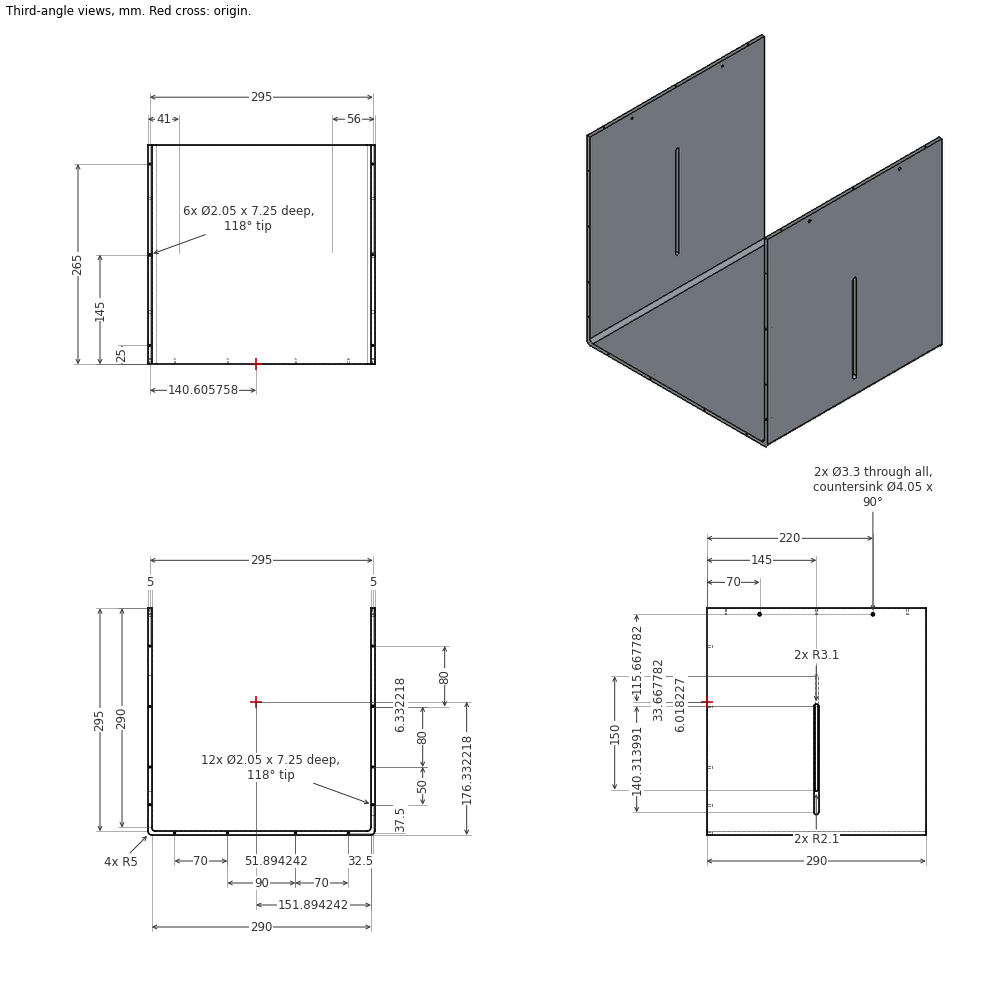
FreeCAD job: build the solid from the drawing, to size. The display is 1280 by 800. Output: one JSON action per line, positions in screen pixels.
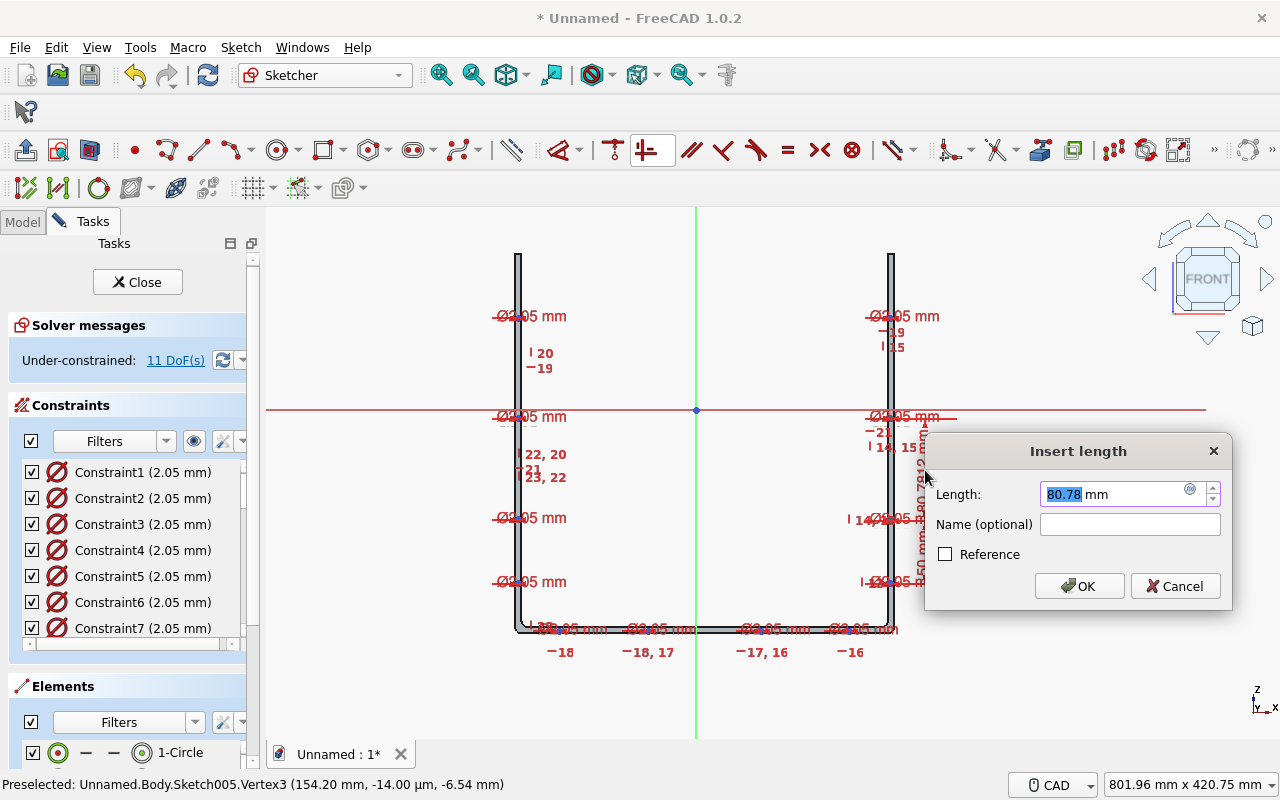
{"action": "type", "text": "80"}
{"action": "key", "text": "Return"}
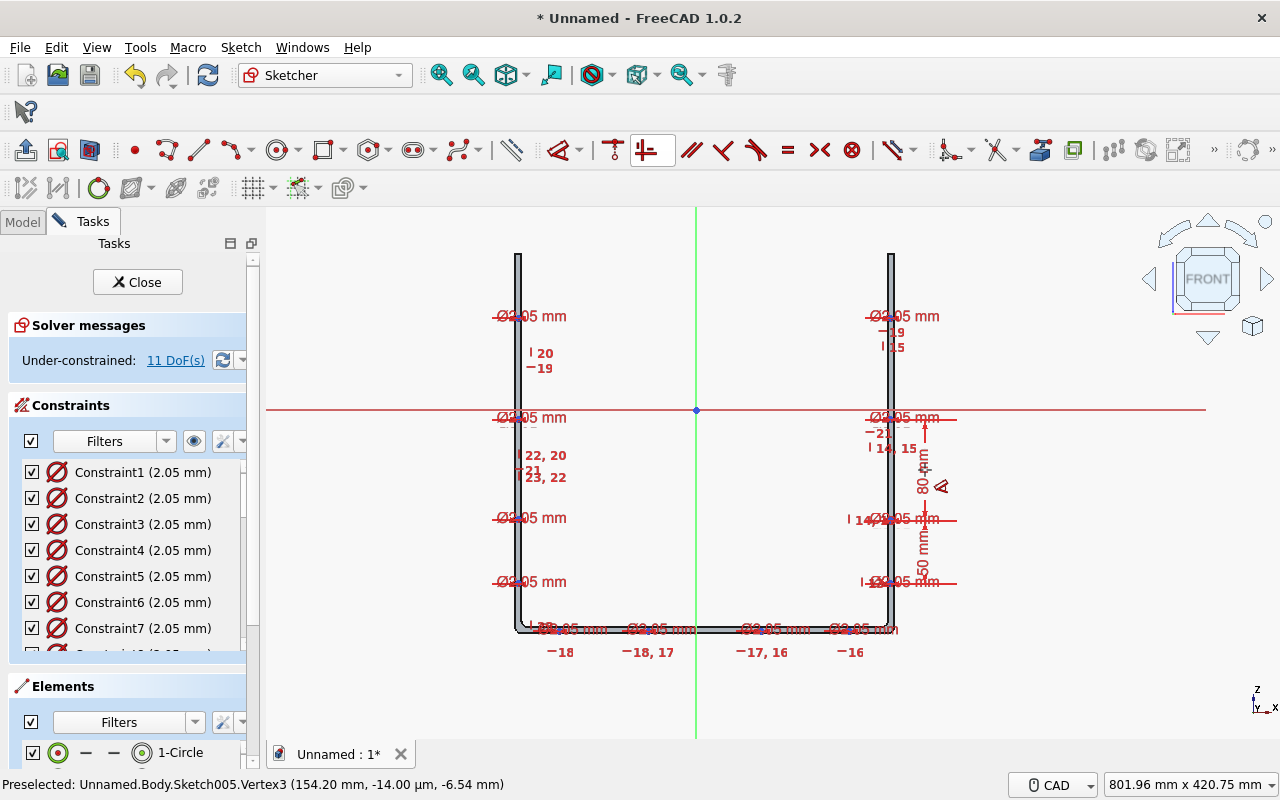
{"action": "left_click", "coordinate": [891, 420]}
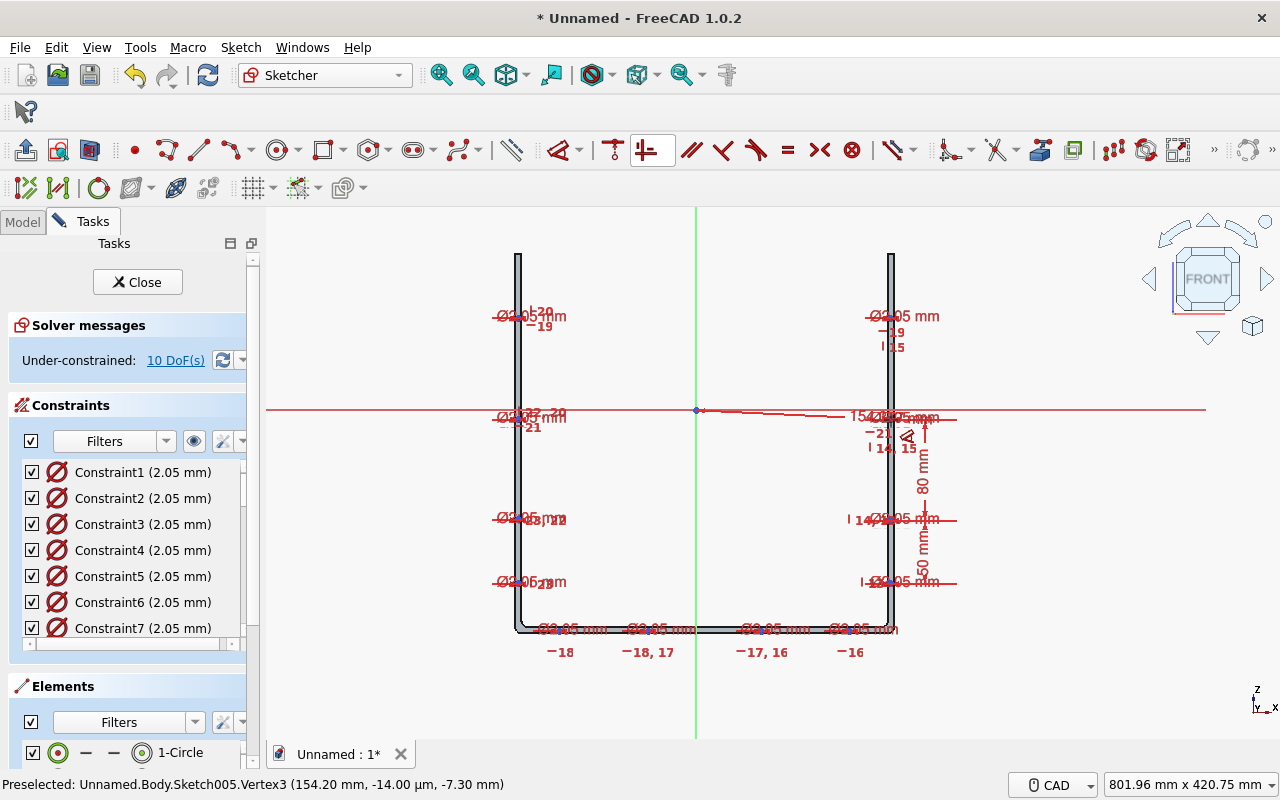
{"action": "left_click", "coordinate": [891, 318]}
{"action": "left_click", "coordinate": [925, 369]}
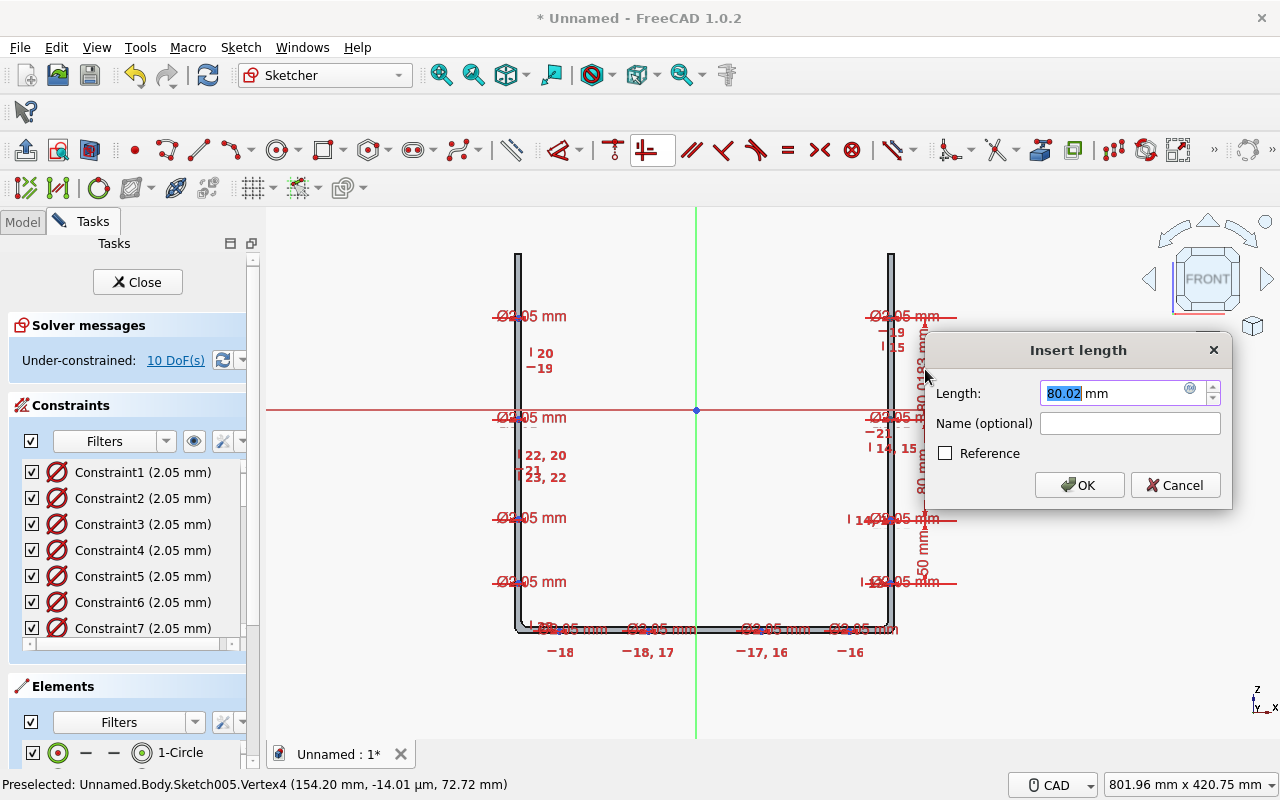
{"action": "type", "text": "80"}
{"action": "key", "text": "Return"}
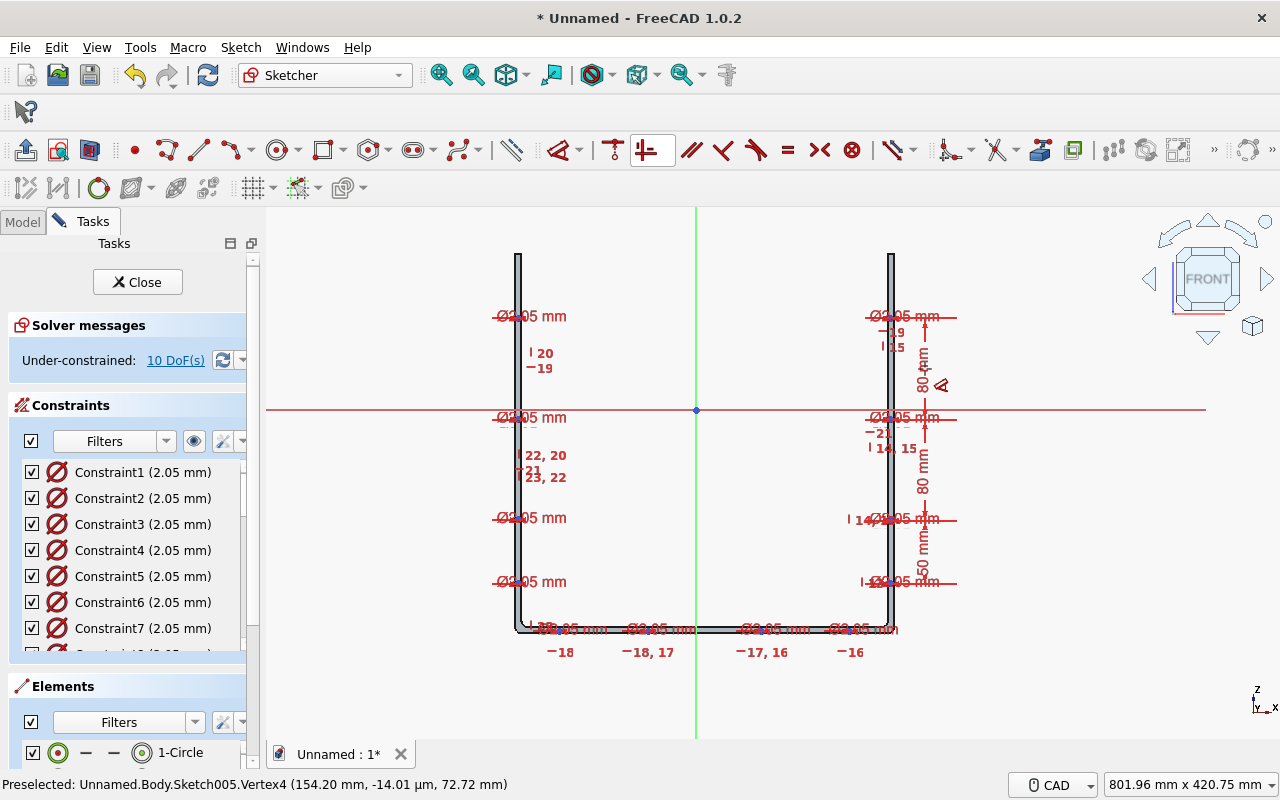
{"action": "left_click", "coordinate": [850, 631]}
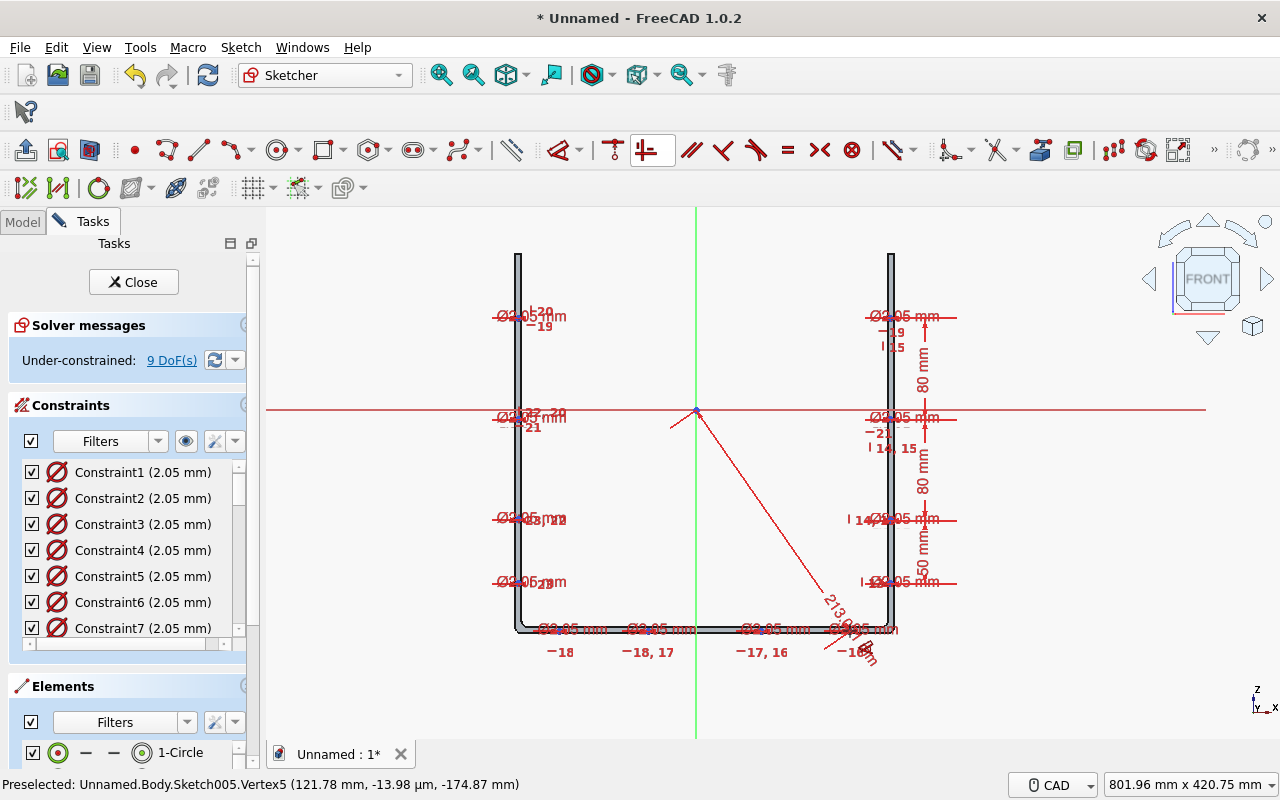
{"action": "left_click", "coordinate": [762, 631]}
{"action": "left_click", "coordinate": [806, 665]}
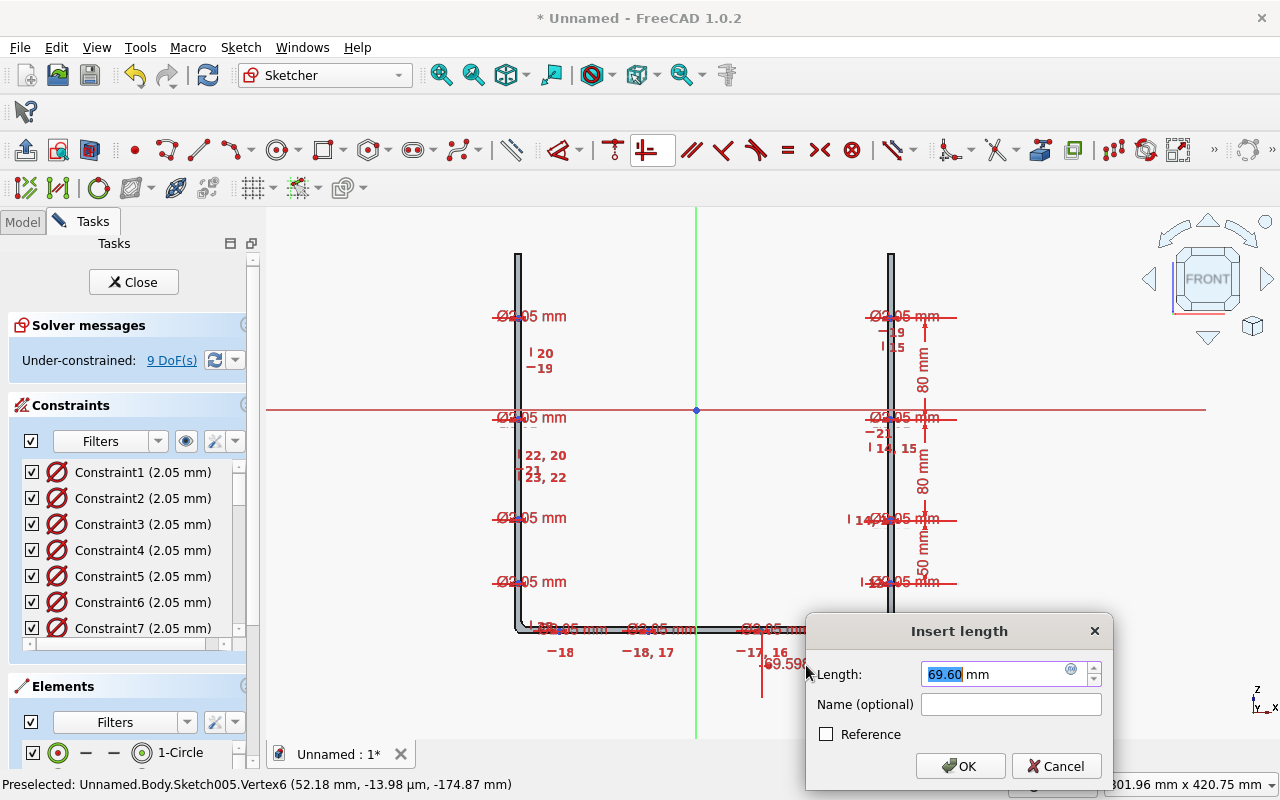
{"action": "type", "text": "70"}
{"action": "key", "text": "Return"}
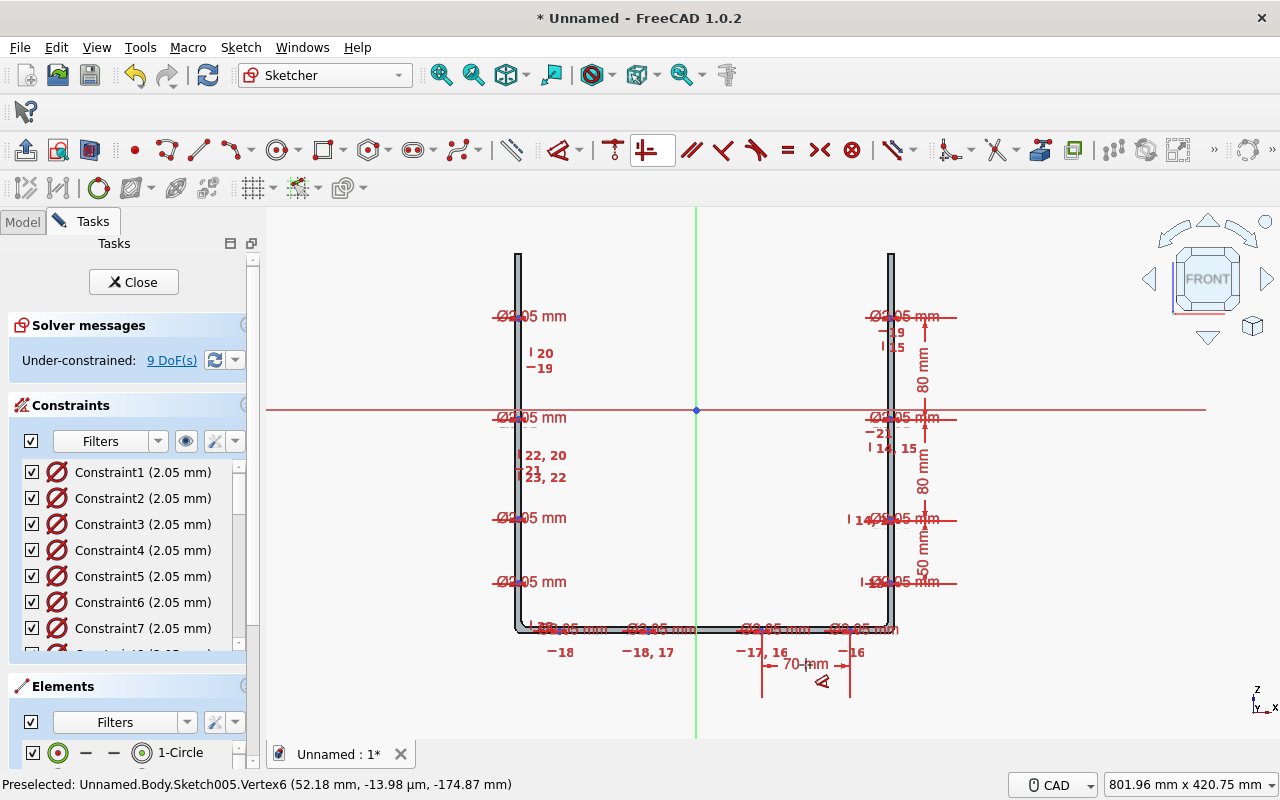
{"action": "left_click", "coordinate": [762, 631]}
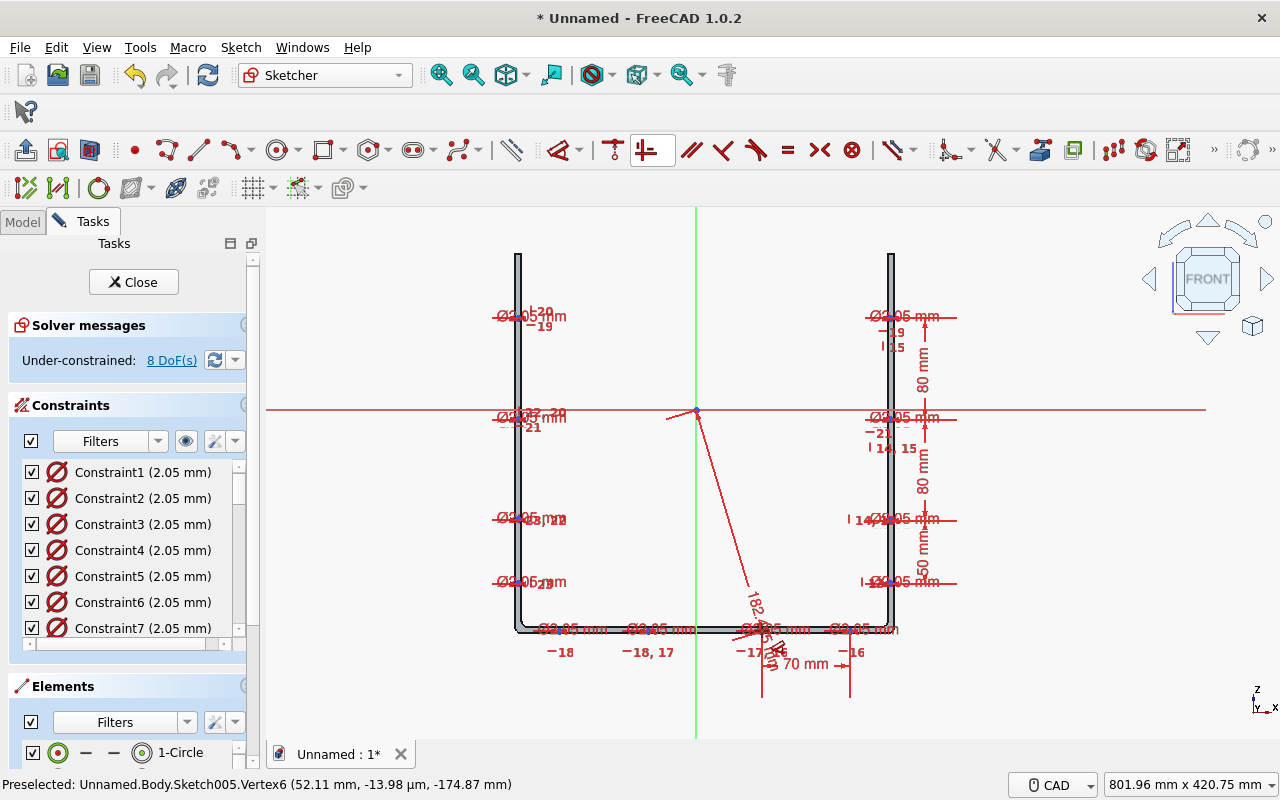
{"action": "left_click", "coordinate": [648, 631]}
{"action": "left_click", "coordinate": [679, 665]}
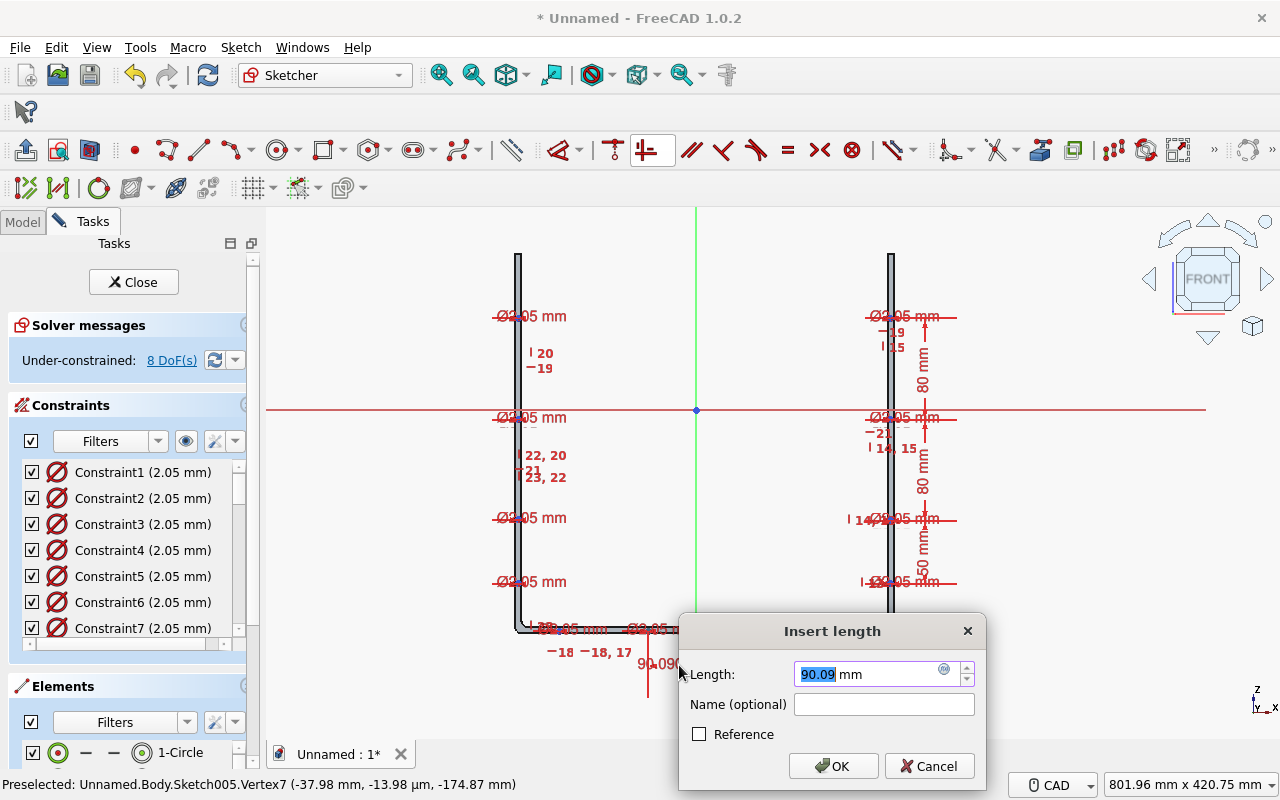
{"action": "type", "text": "90"}
{"action": "key", "text": "Return"}